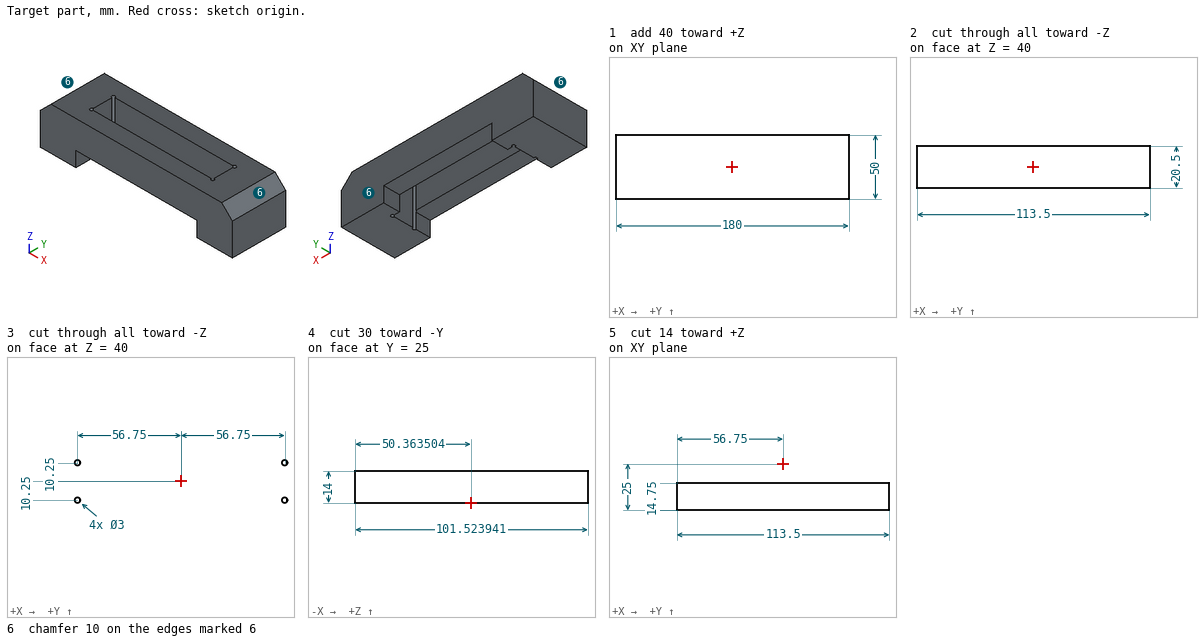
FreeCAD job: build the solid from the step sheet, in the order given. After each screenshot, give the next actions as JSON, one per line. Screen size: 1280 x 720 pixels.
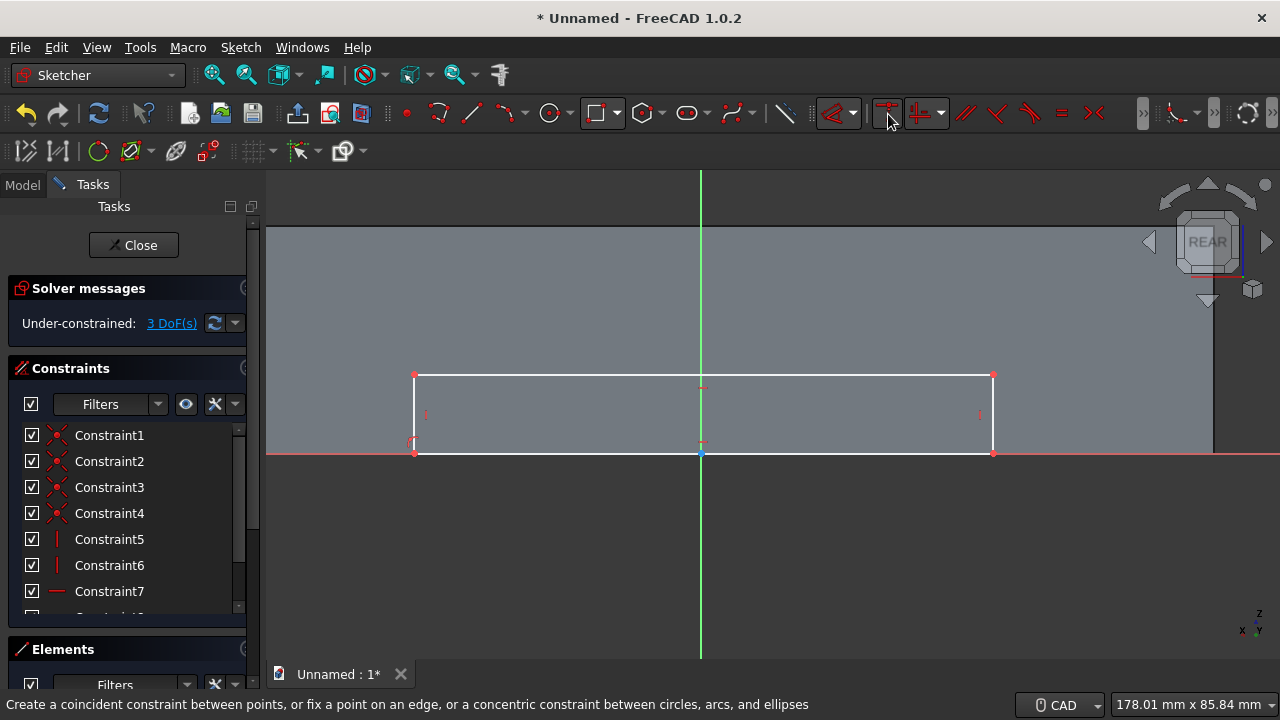
{"action": "left_click", "coordinate": [414, 399]}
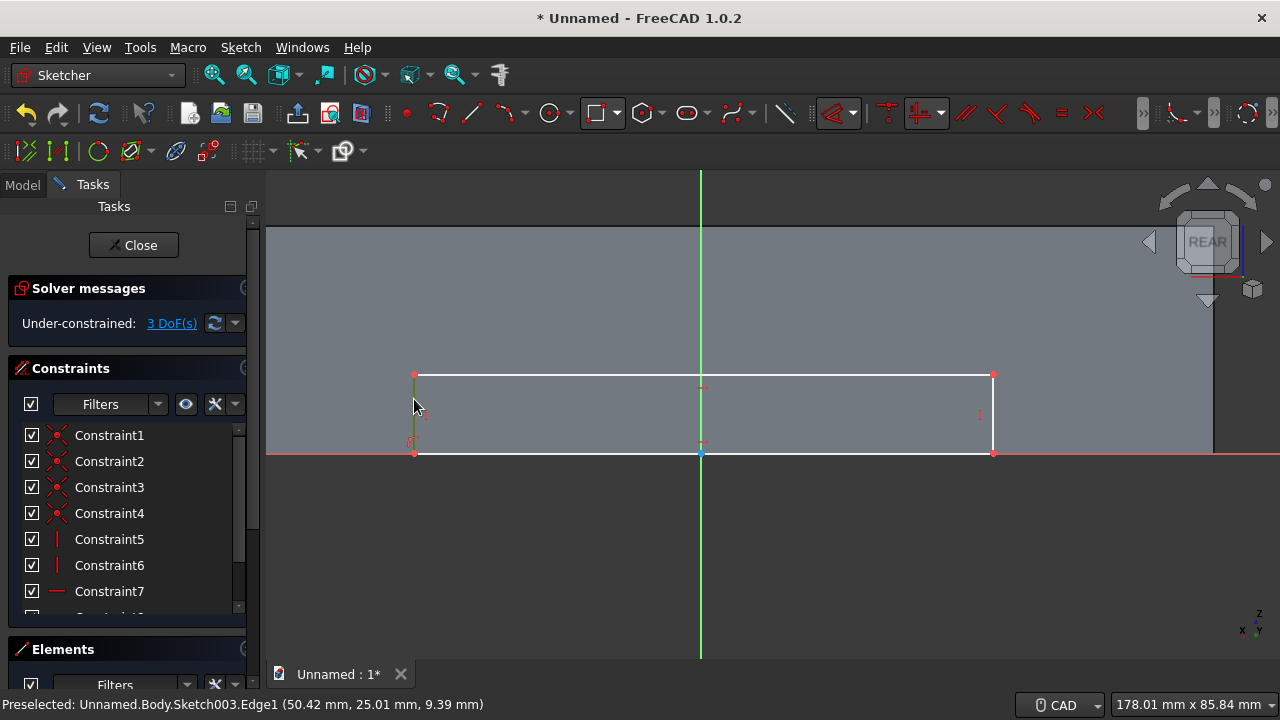
{"action": "left_click", "coordinate": [856, 114]}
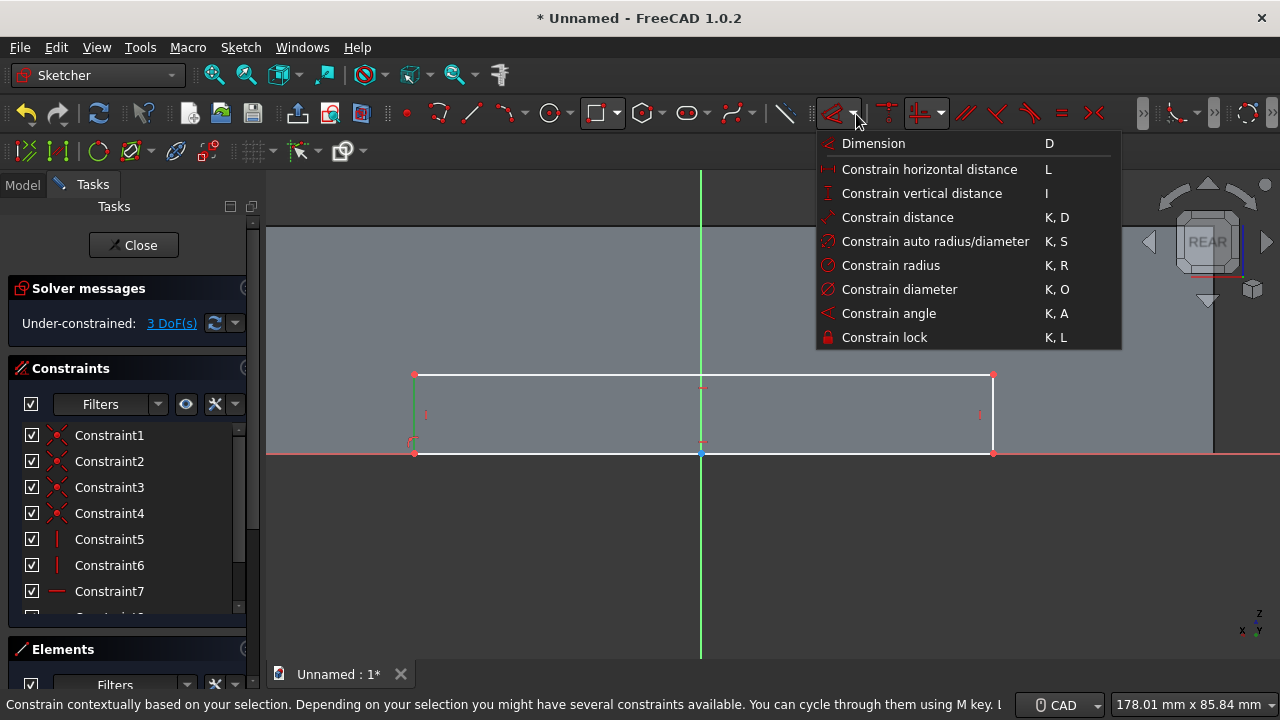
{"action": "left_click", "coordinate": [969, 193]}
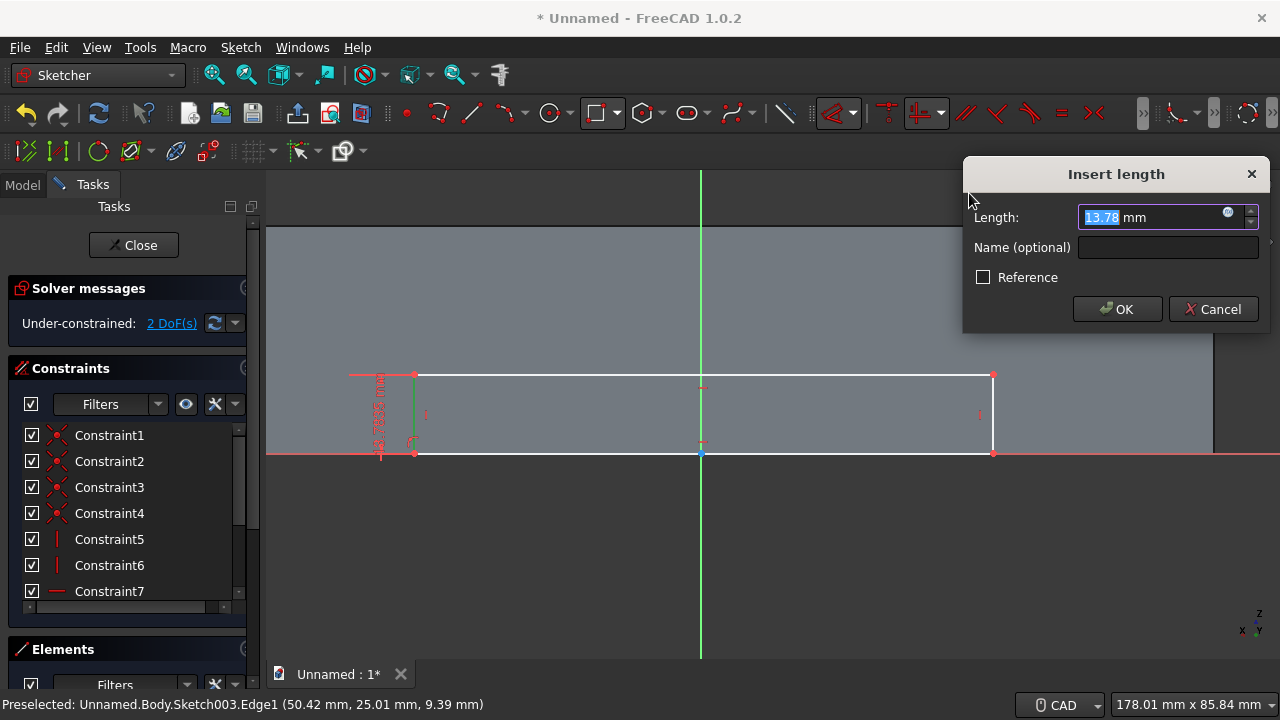
{"action": "type", "text": "14"}
{"action": "key", "text": "Return"}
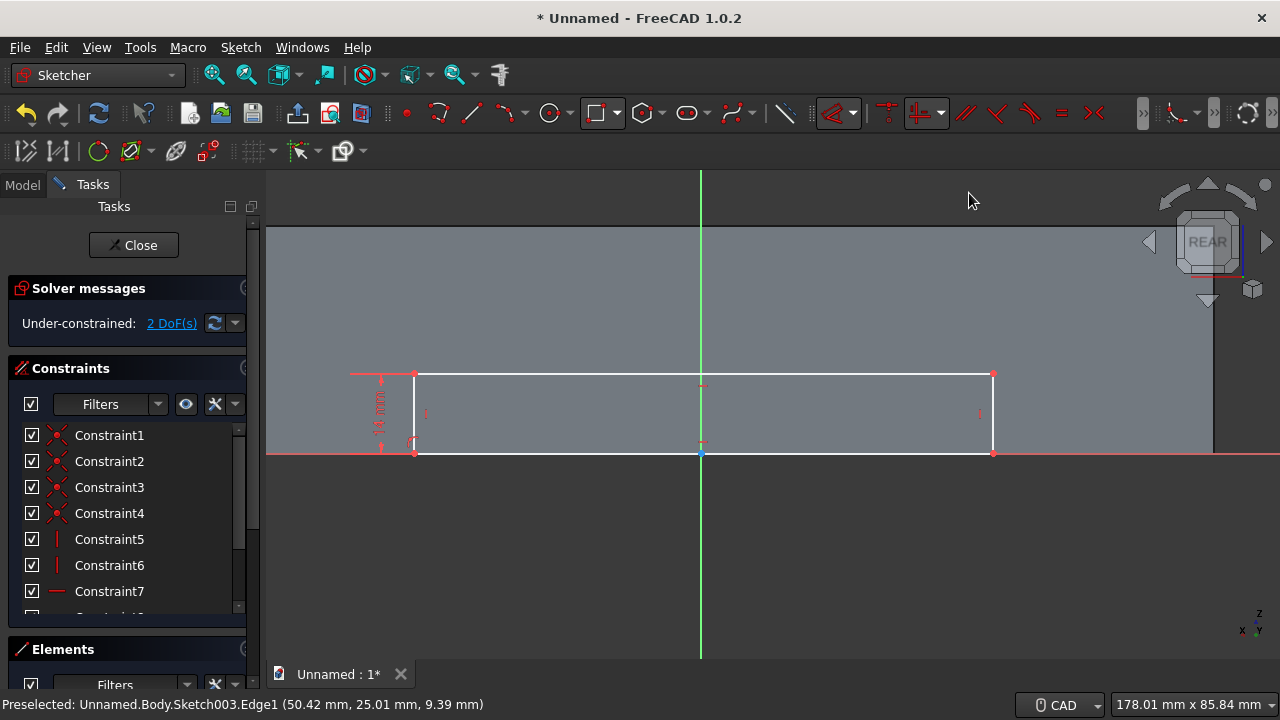
{"action": "left_click", "coordinate": [588, 454]}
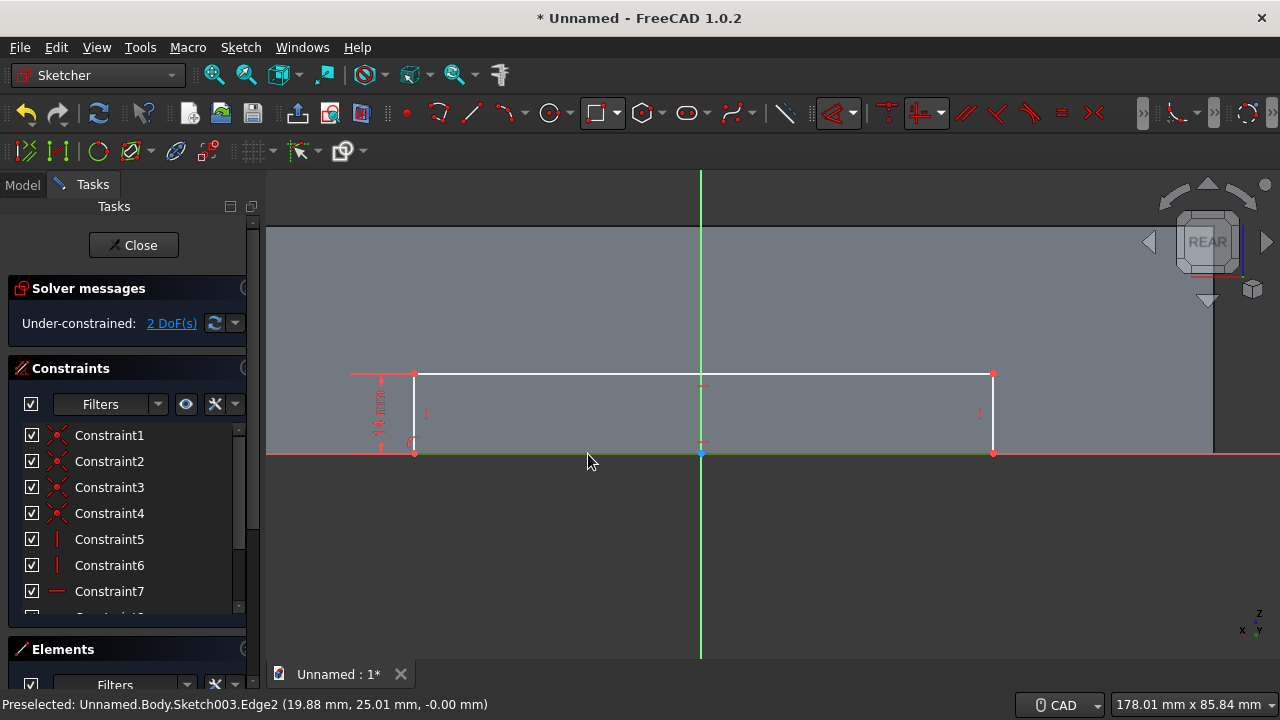
{"action": "left_click", "coordinate": [856, 114]}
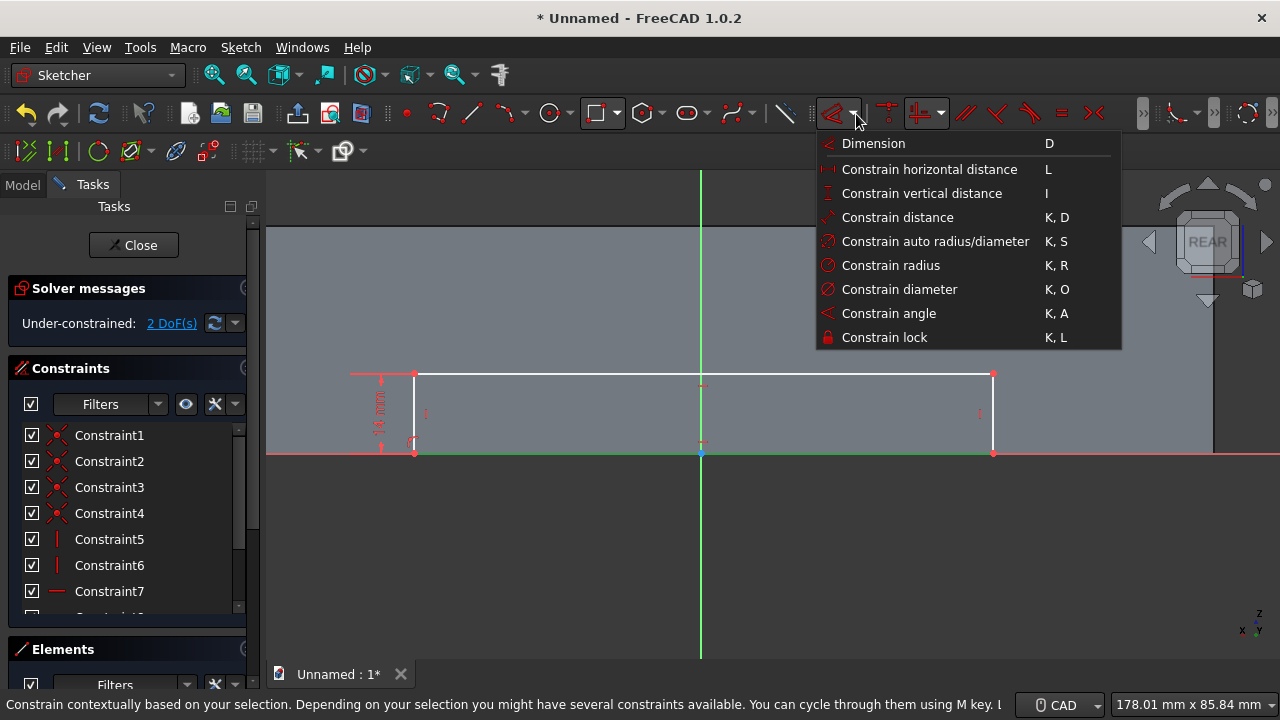
{"action": "left_click", "coordinate": [969, 169]}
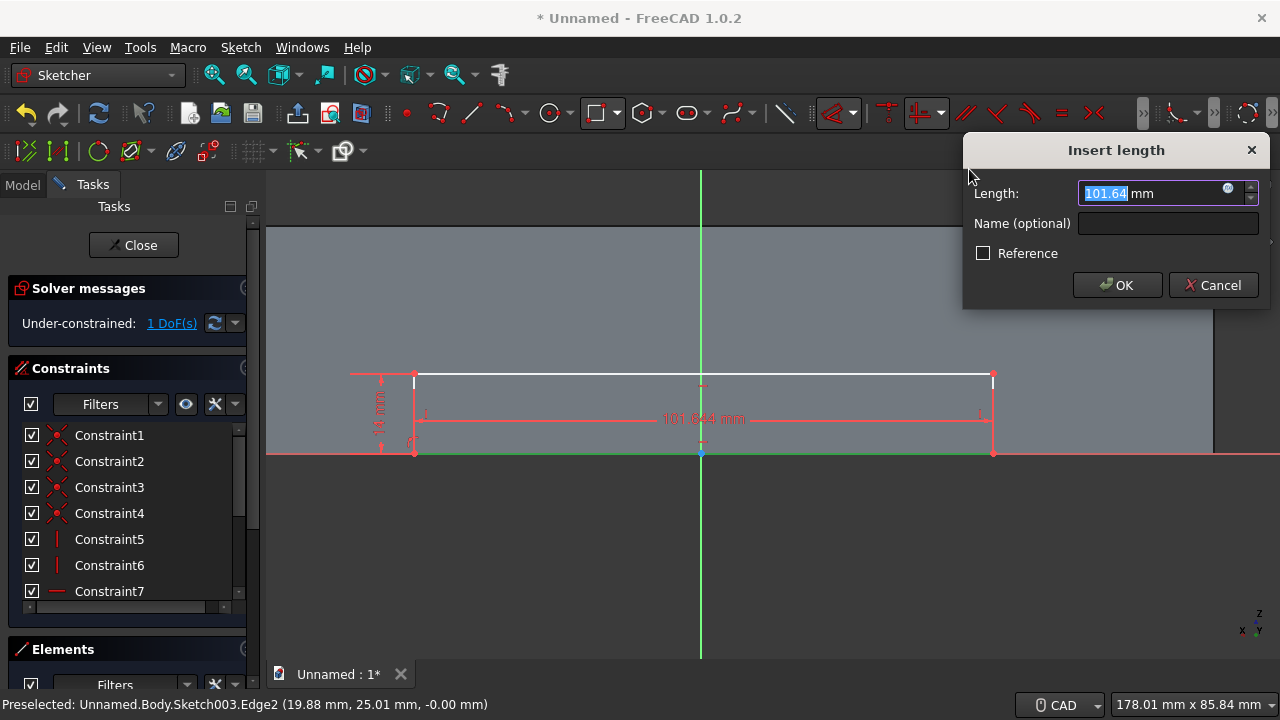
{"action": "type", "text": "101.523941"}
{"action": "key", "text": "Return"}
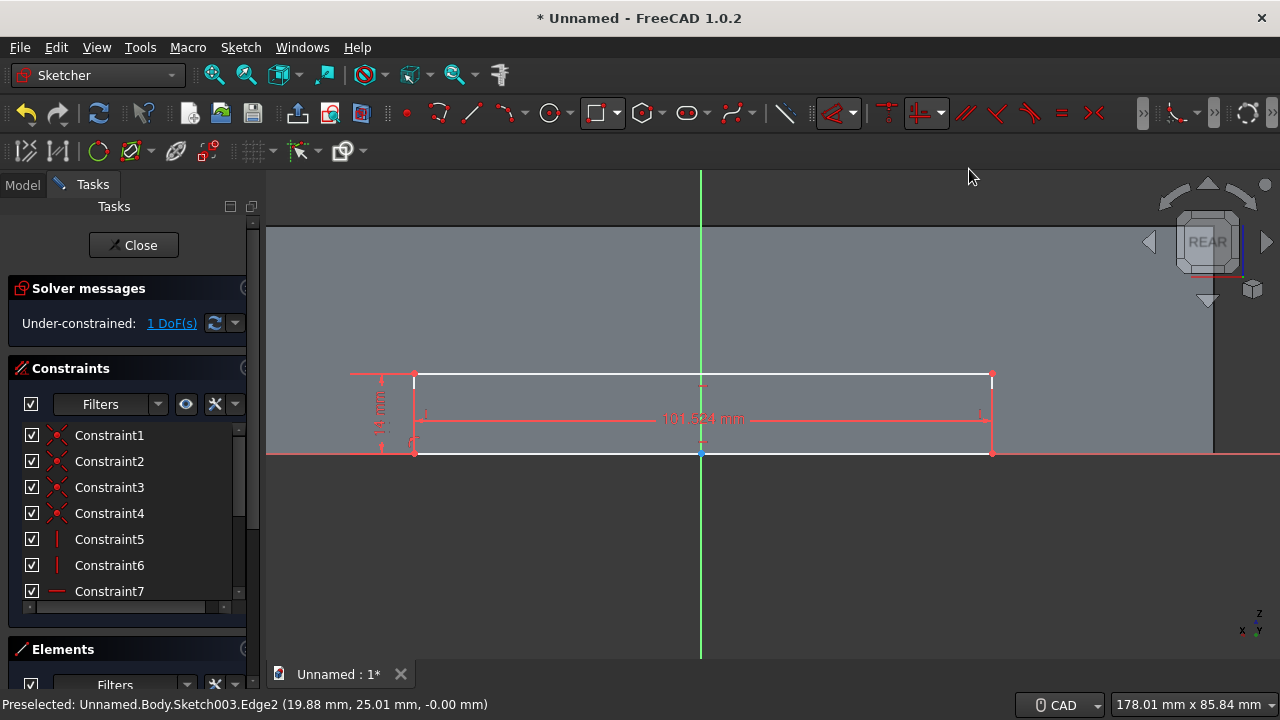
{"action": "left_click", "coordinate": [414, 374]}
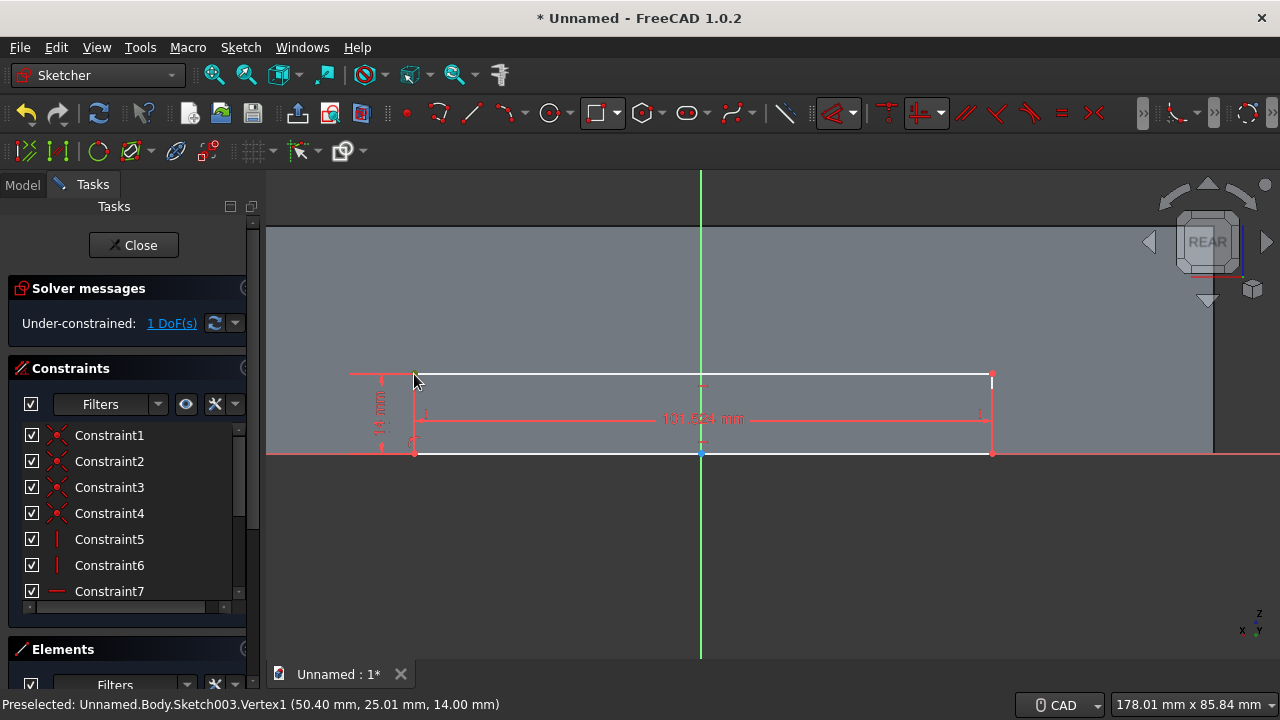
{"action": "key", "text": "l"}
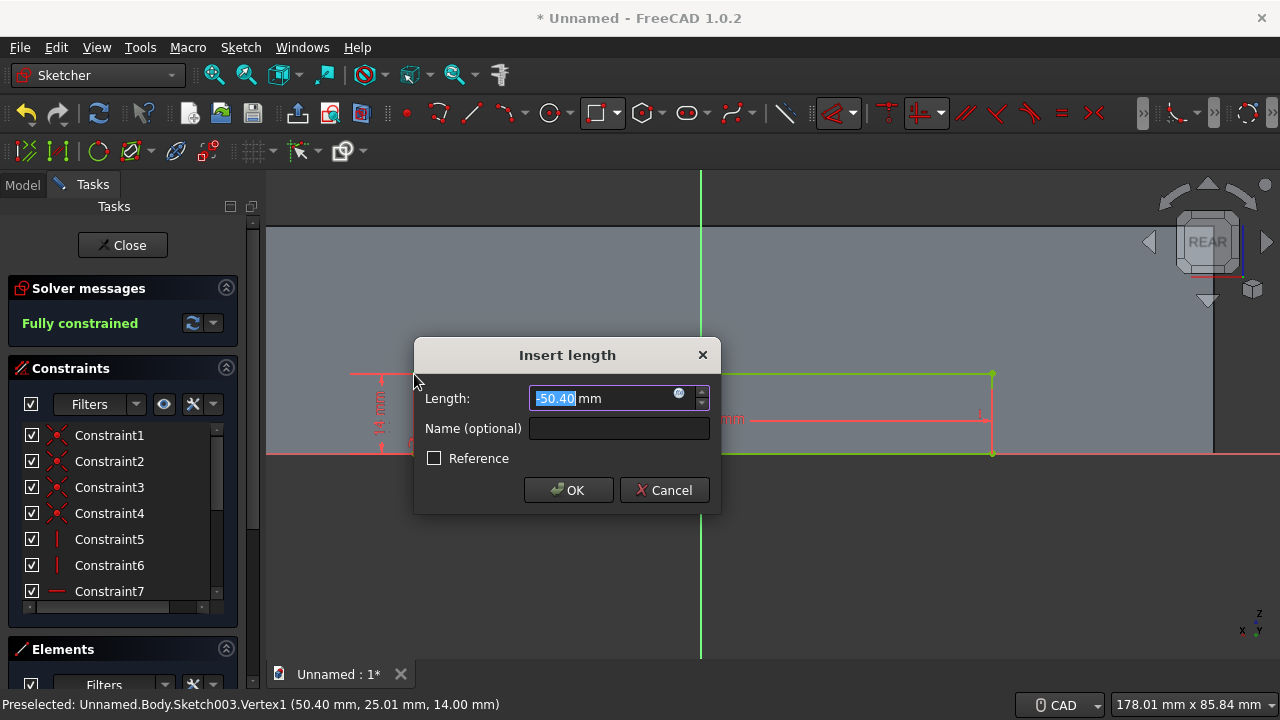
{"action": "type", "text": "-50.363504"}
{"action": "key", "text": "Return"}